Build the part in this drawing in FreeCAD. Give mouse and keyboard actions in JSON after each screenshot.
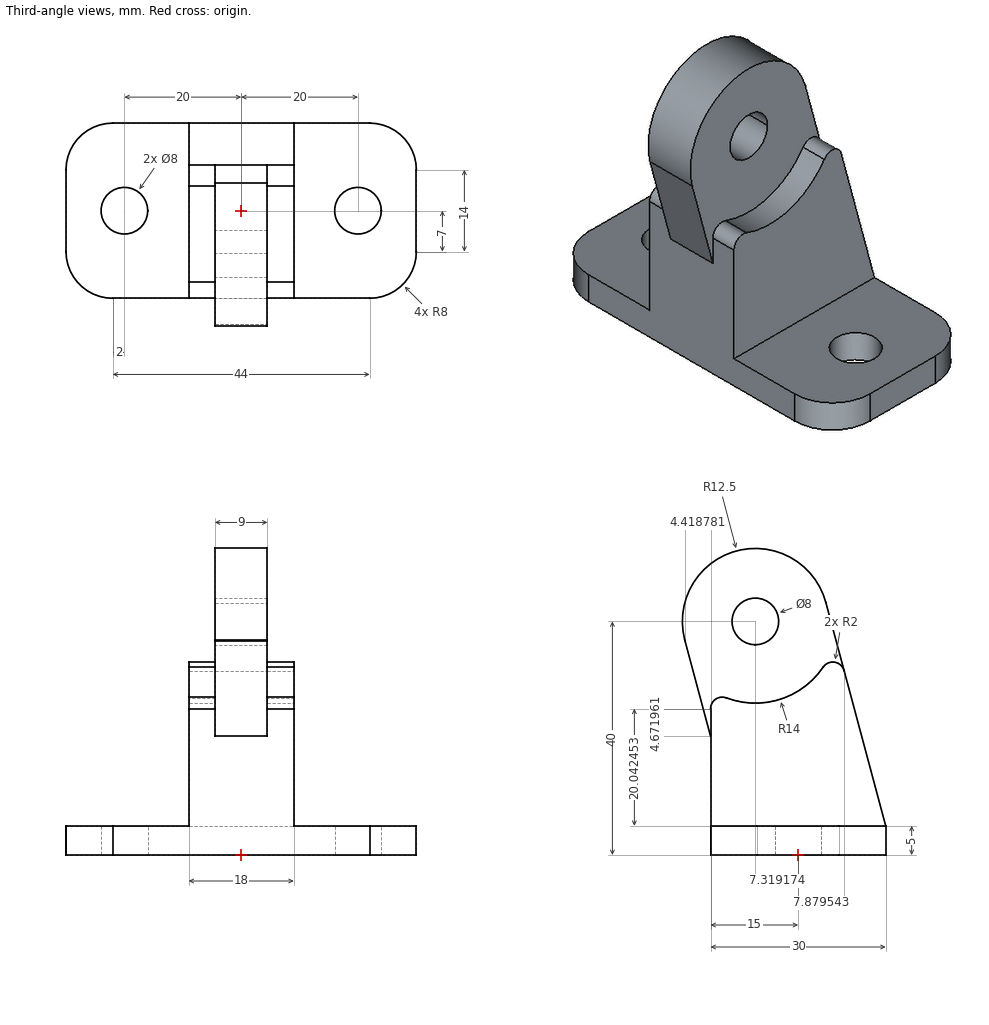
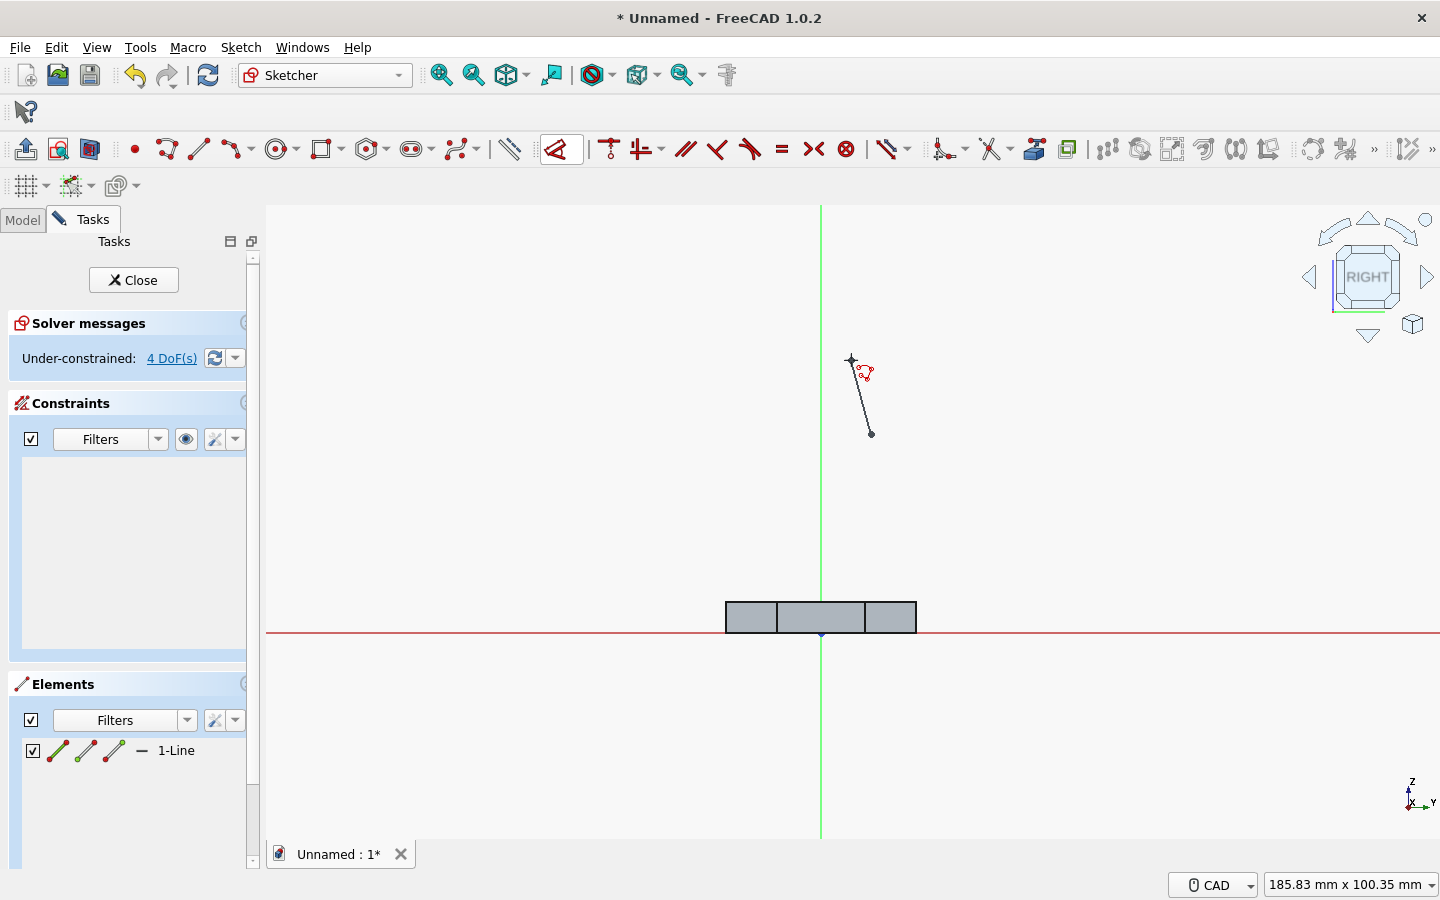
{"action": "left_click", "coordinate": [698, 401]}
{"action": "left_click", "coordinate": [726, 505]}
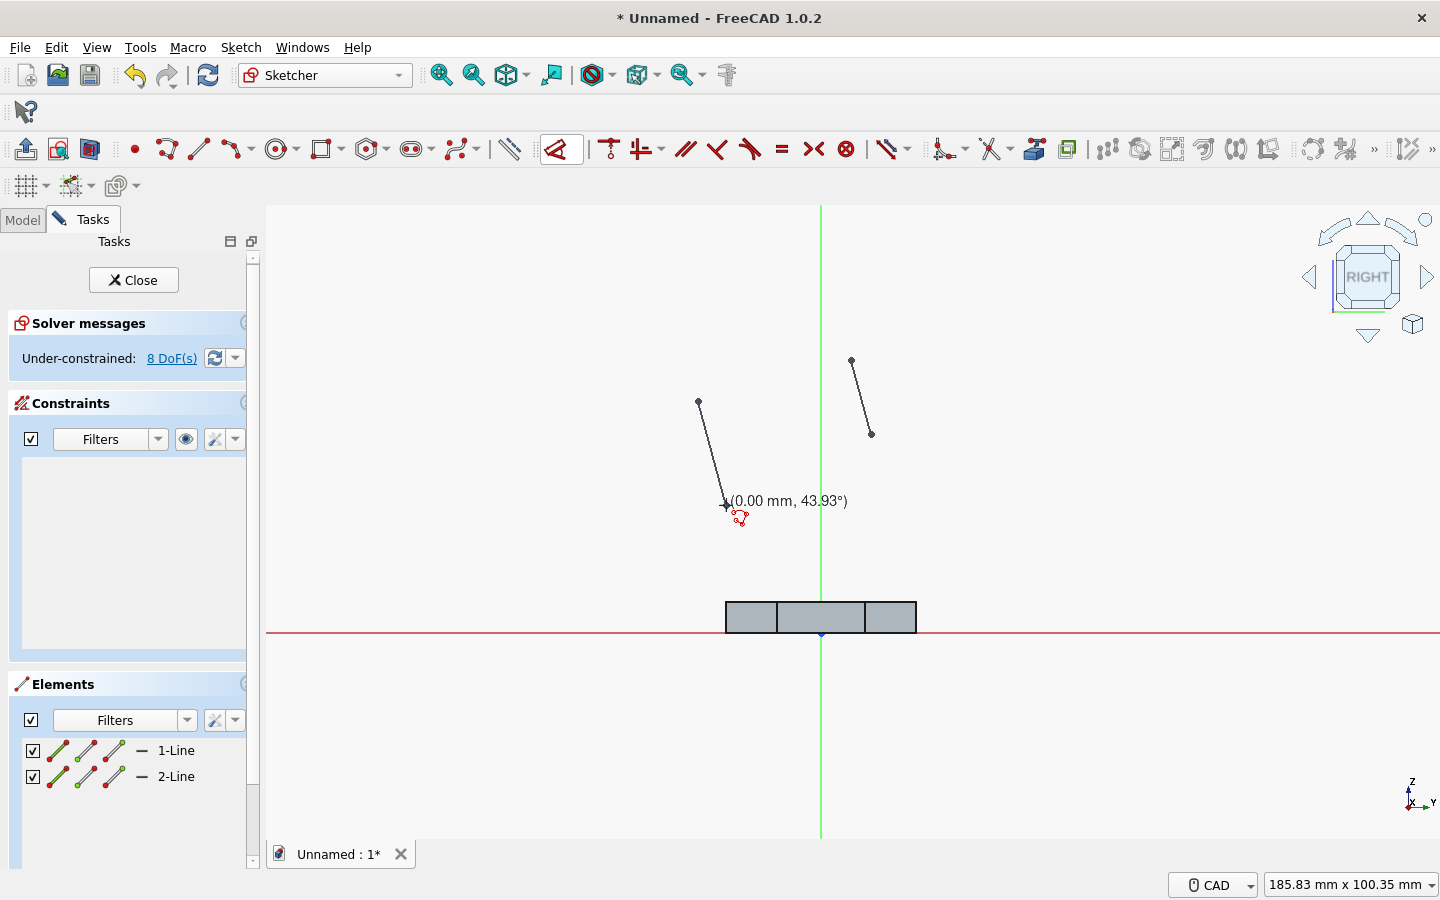
{"action": "scroll", "coordinate": [726, 475], "scroll_direction": "up", "scroll_amount": 4}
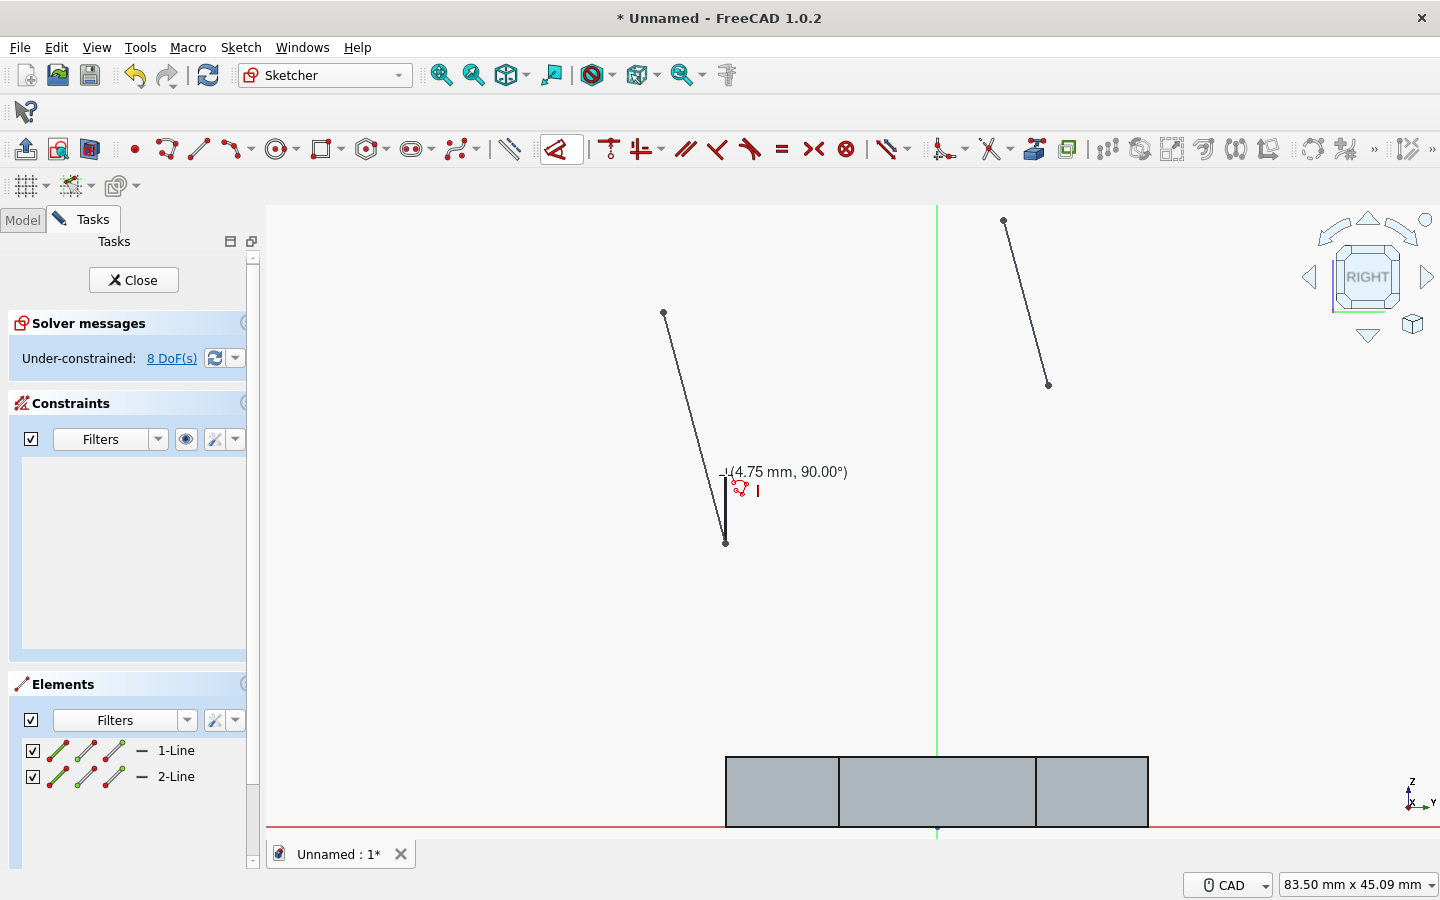
{"action": "left_click", "coordinate": [726, 475]}
{"action": "right_click", "coordinate": [726, 475]}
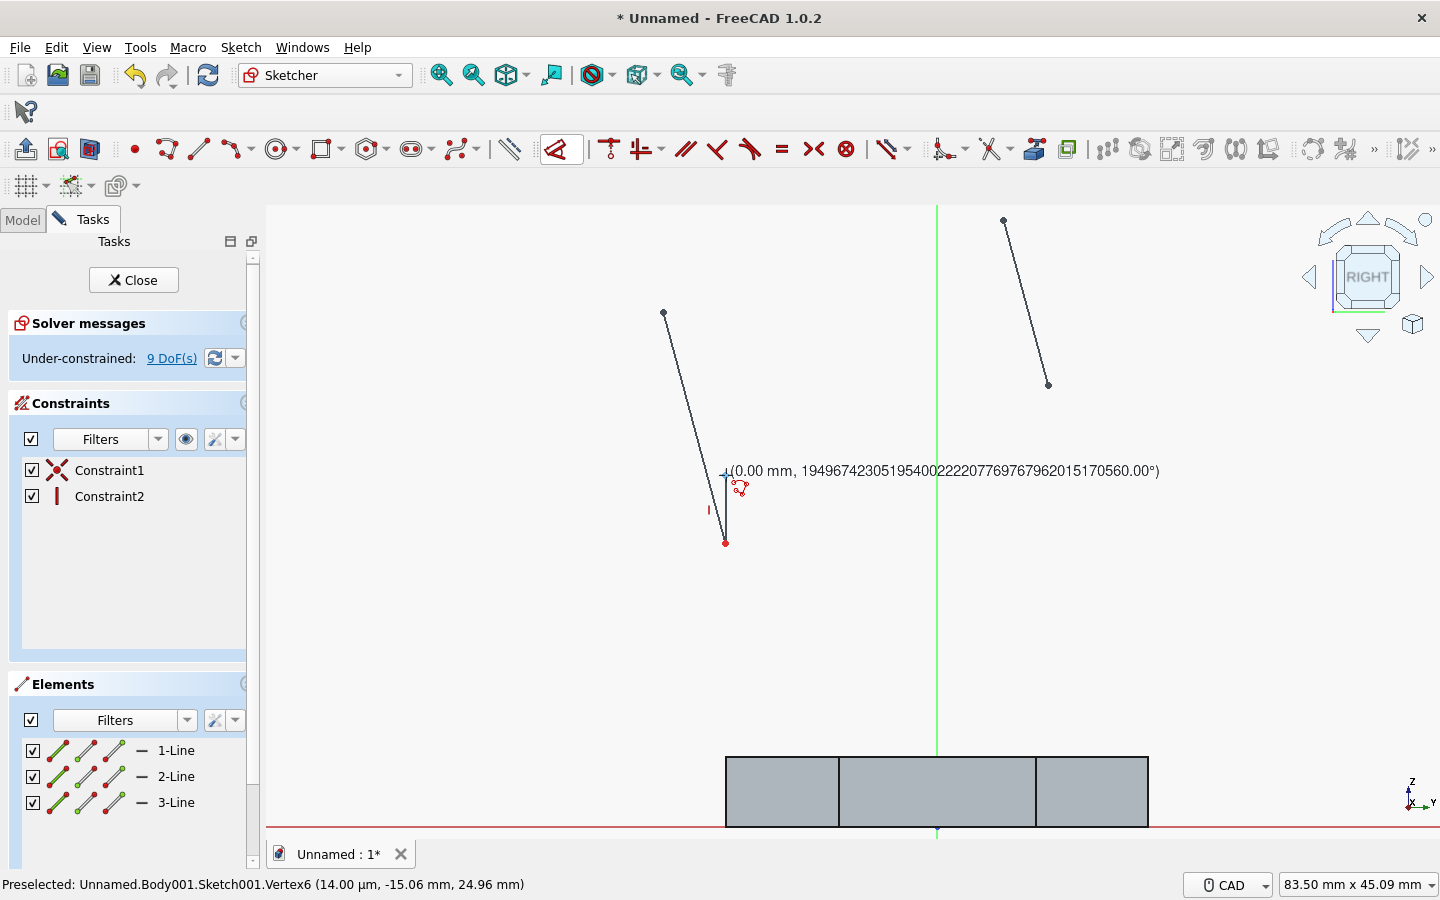
{"action": "key", "text": "g 3 a"}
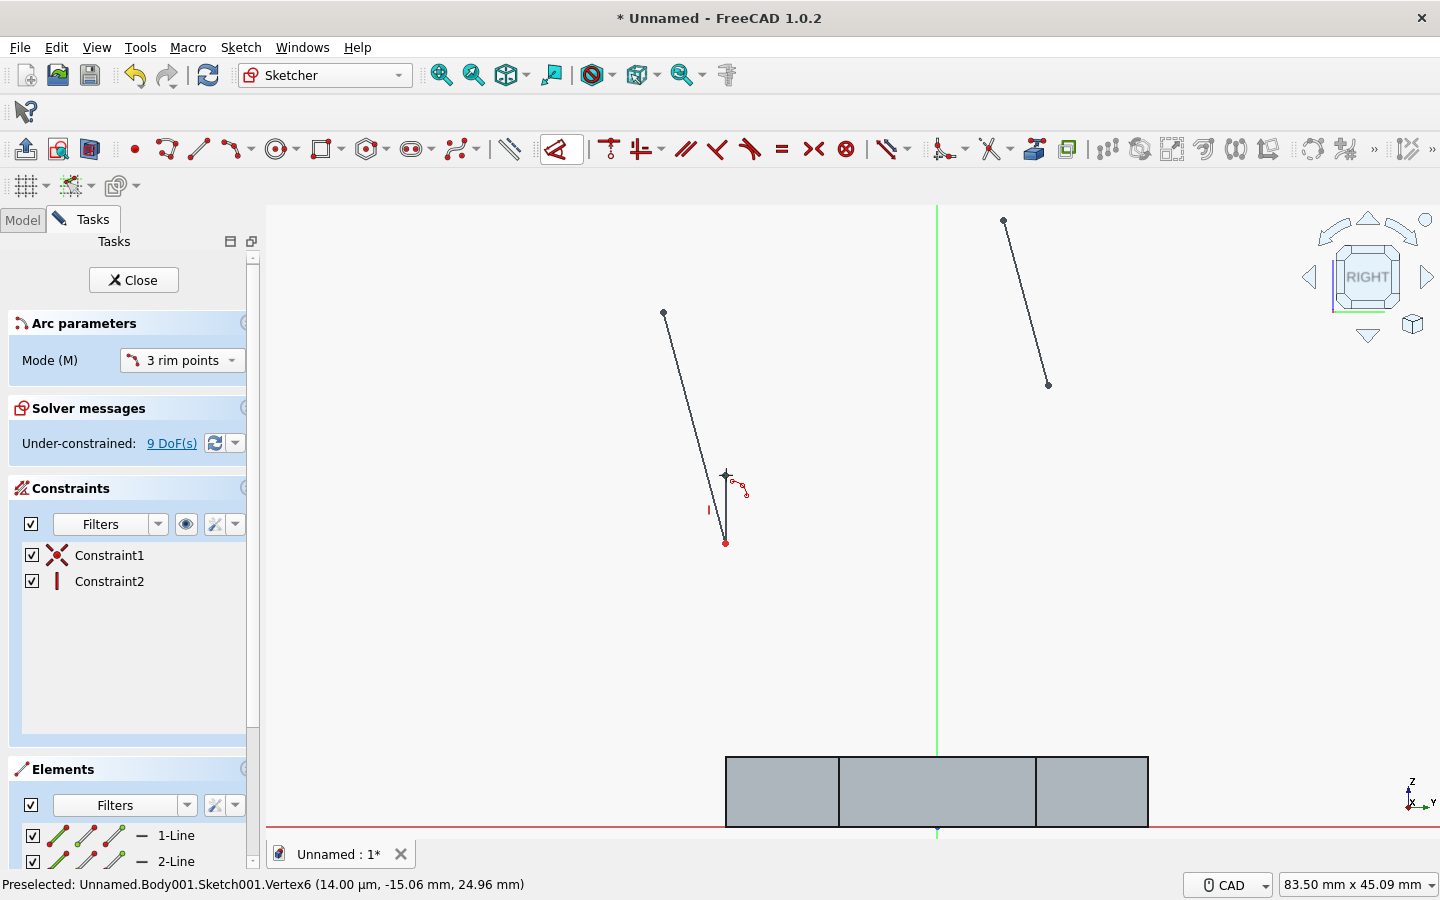
{"action": "scroll", "coordinate": [697, 596], "scroll_direction": "down", "scroll_amount": 3}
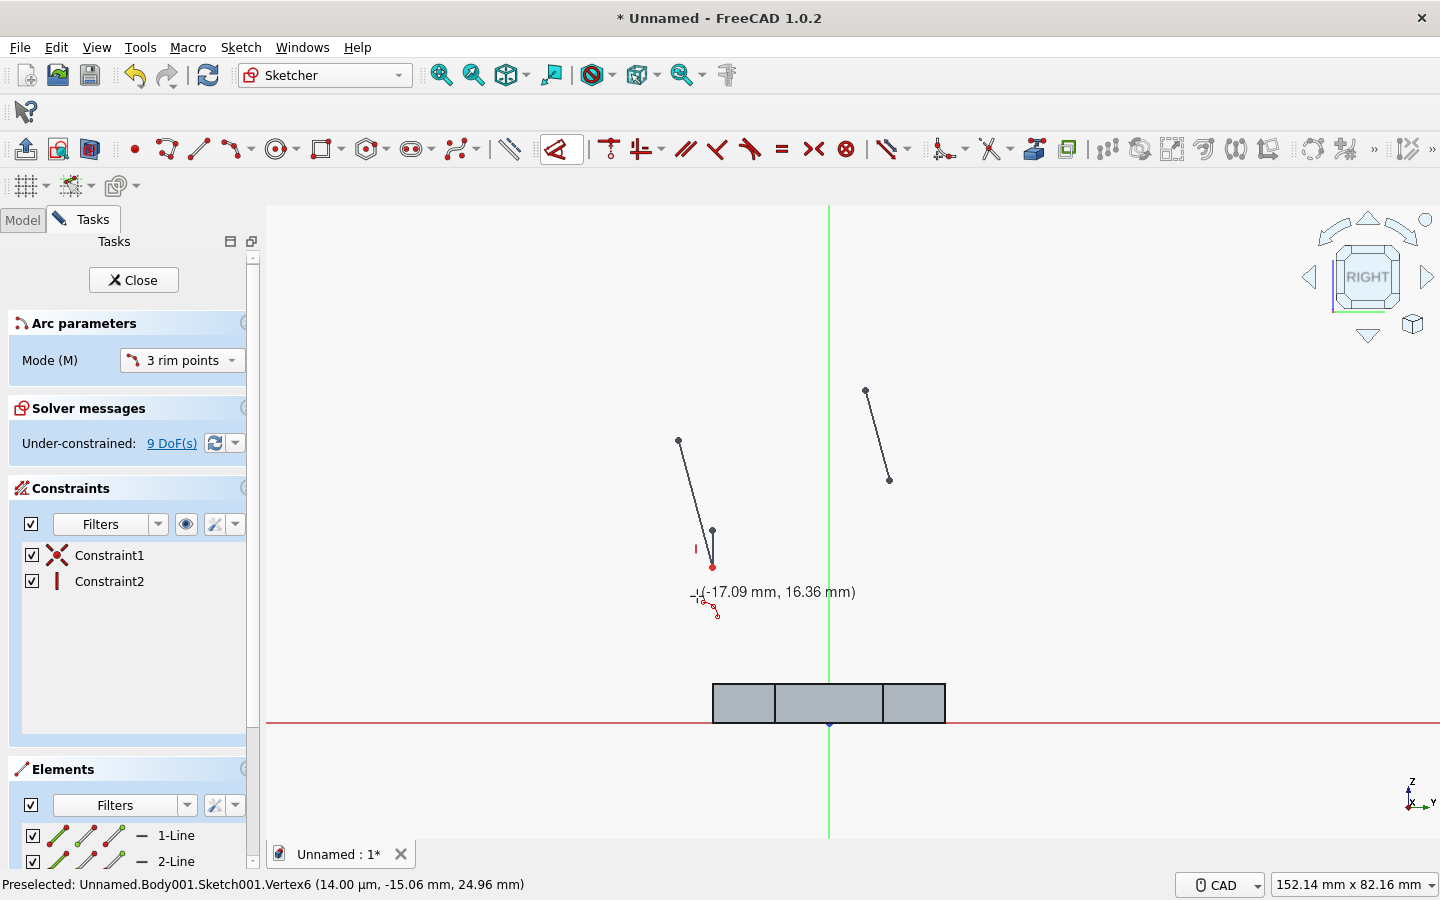
{"action": "left_click", "coordinate": [865, 390]}
{"action": "left_click", "coordinate": [679, 440]}
{"action": "left_click", "coordinate": [748, 321]}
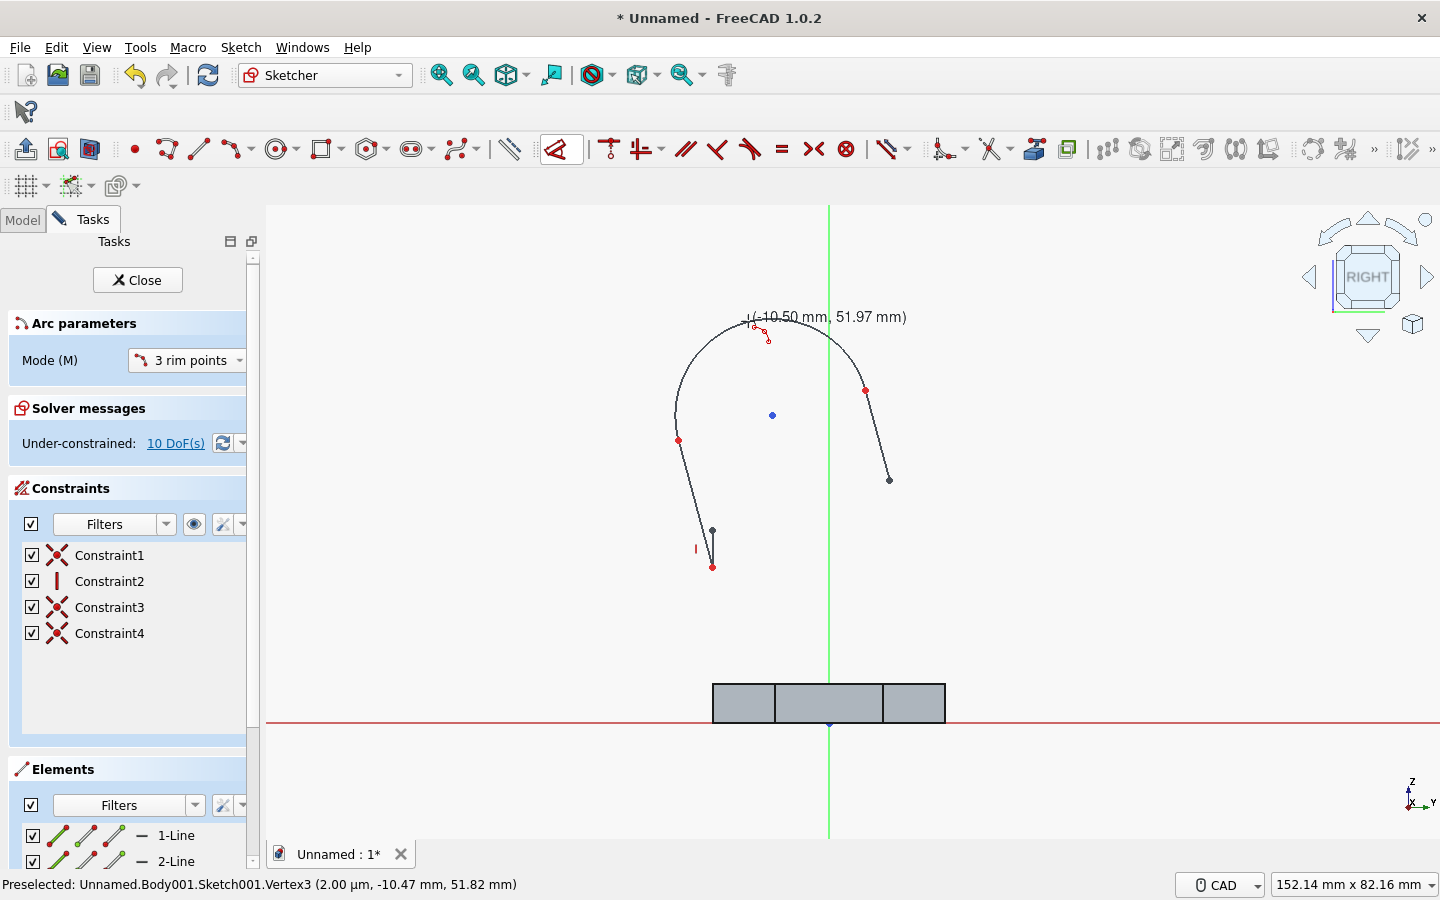
{"action": "scroll", "coordinate": [713, 530], "scroll_direction": "up", "scroll_amount": 3}